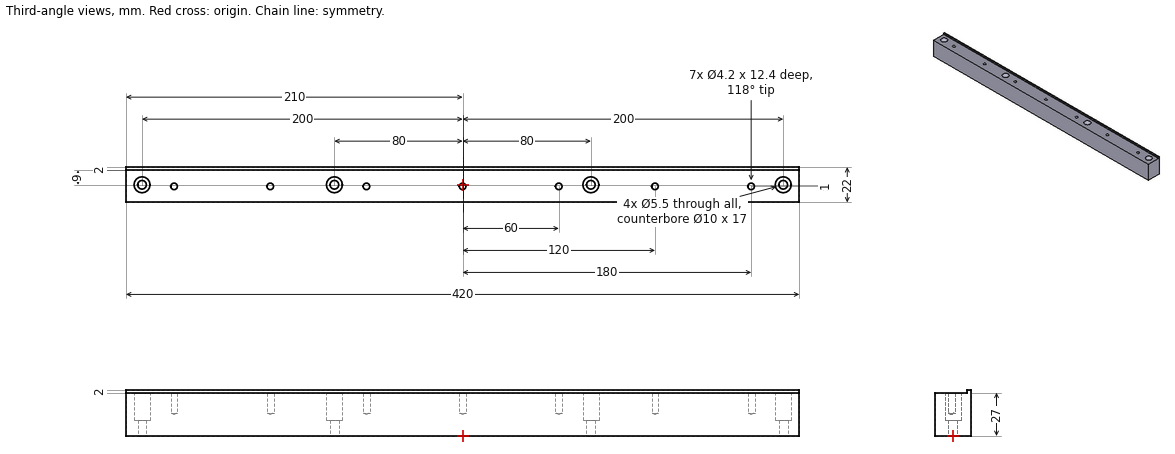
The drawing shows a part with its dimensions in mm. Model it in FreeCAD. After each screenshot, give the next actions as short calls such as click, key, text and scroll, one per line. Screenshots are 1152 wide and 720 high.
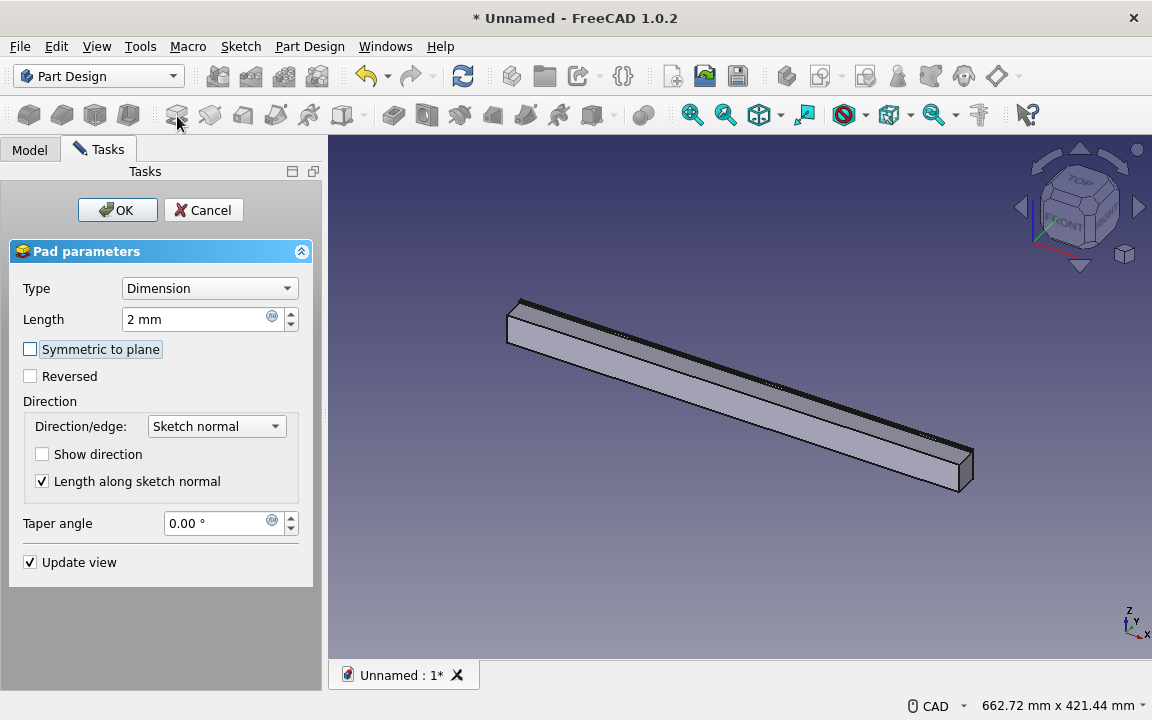
click(118, 210)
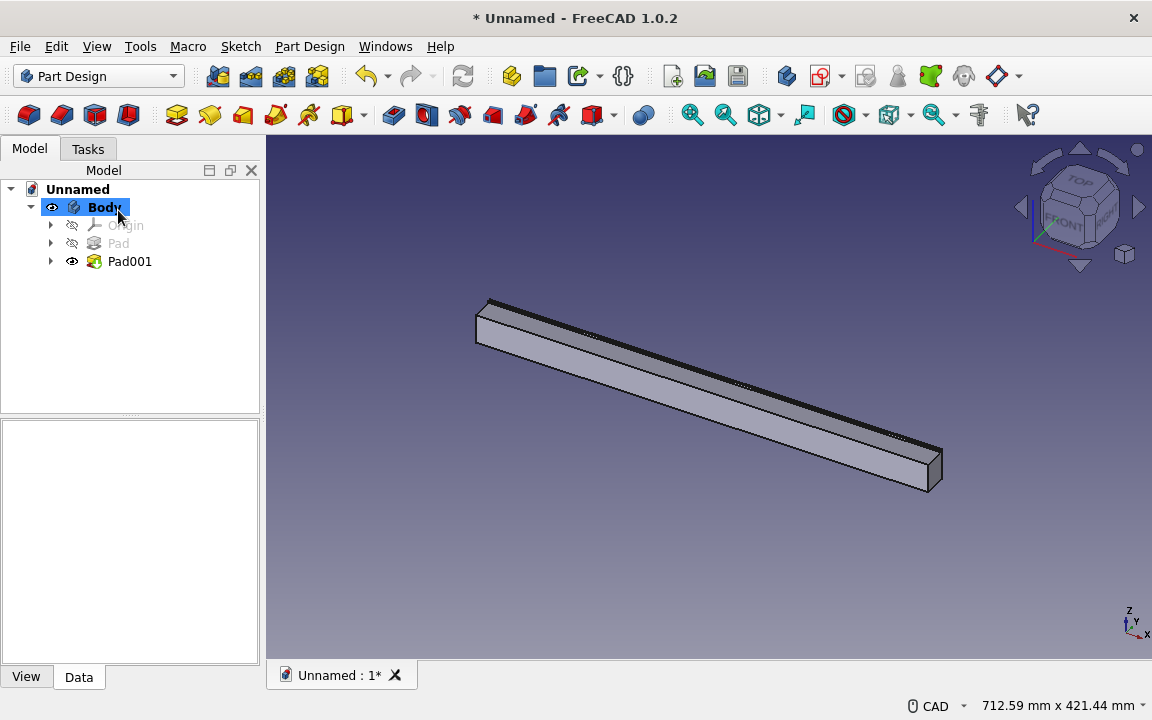
key(0)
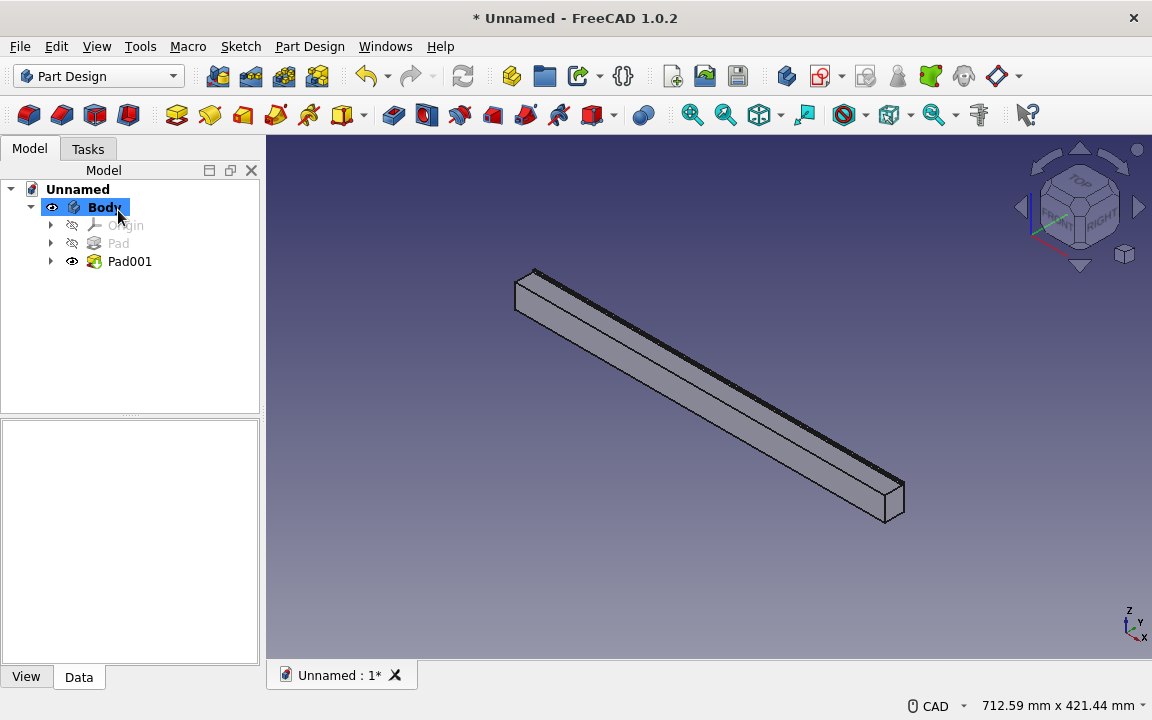
click(762, 413)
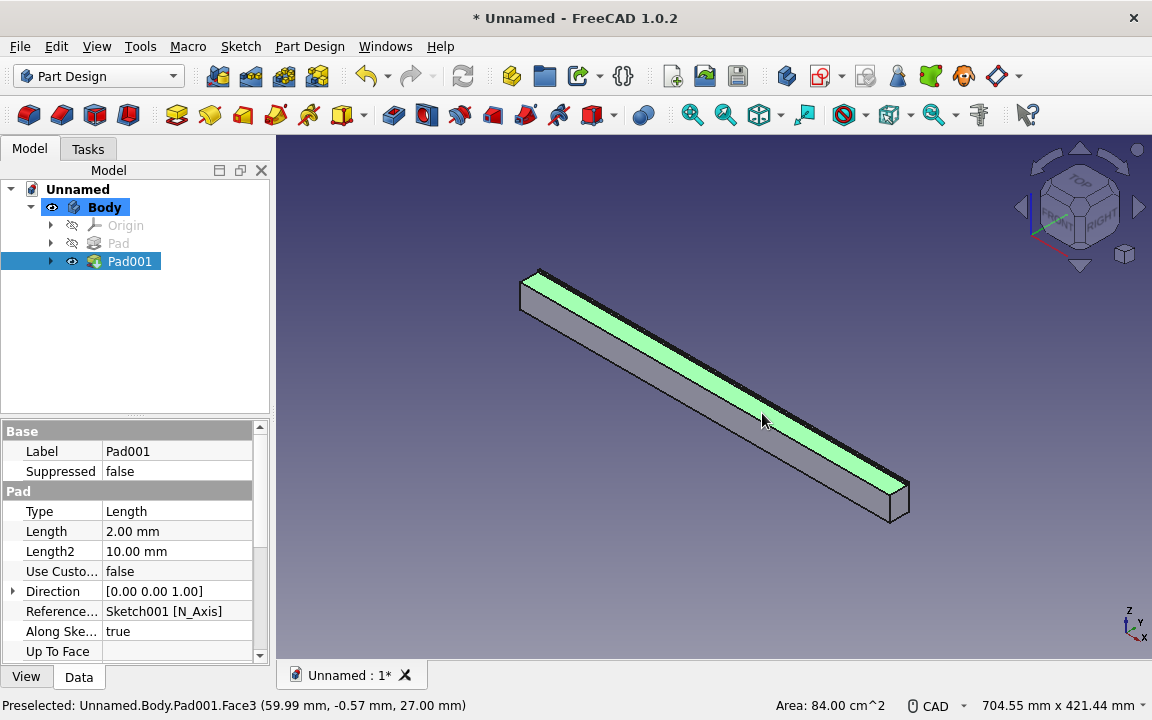
click(820, 76)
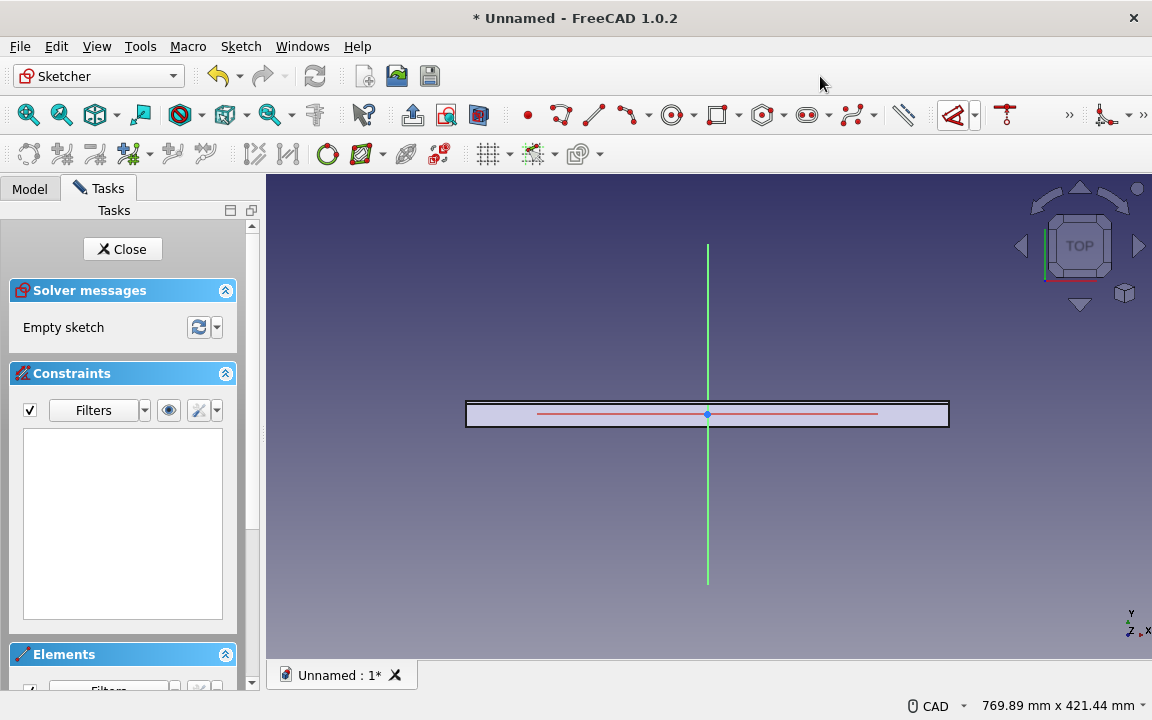
key(q)
key(s)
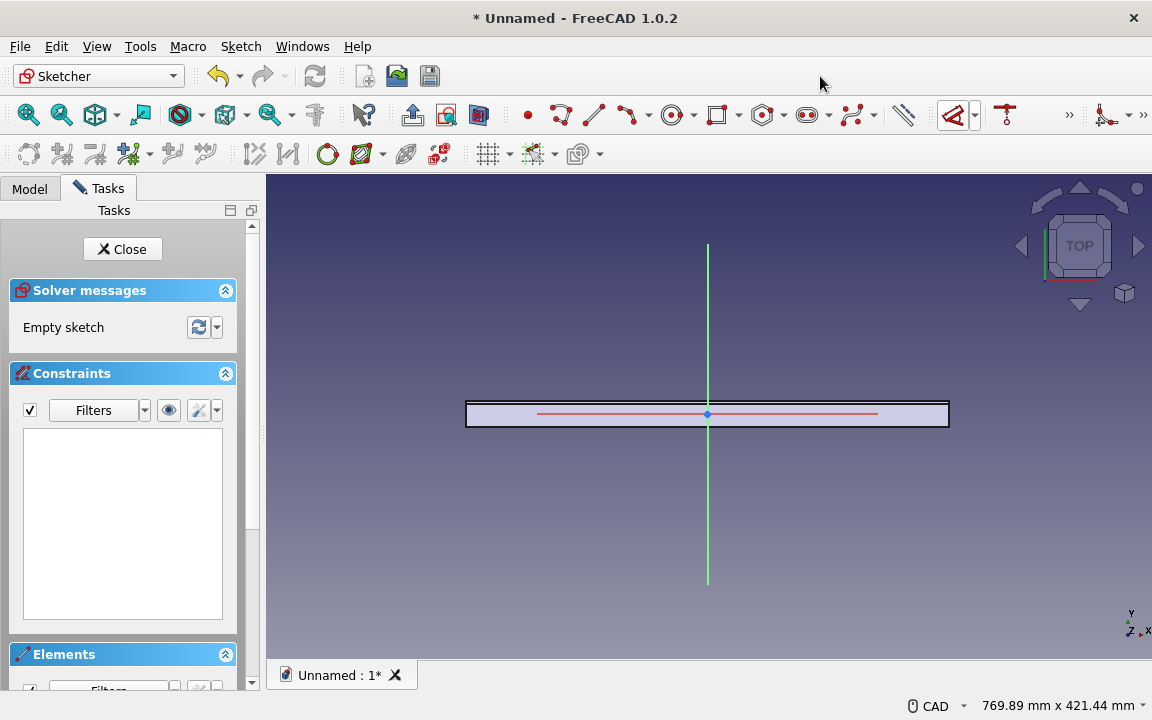
click(672, 116)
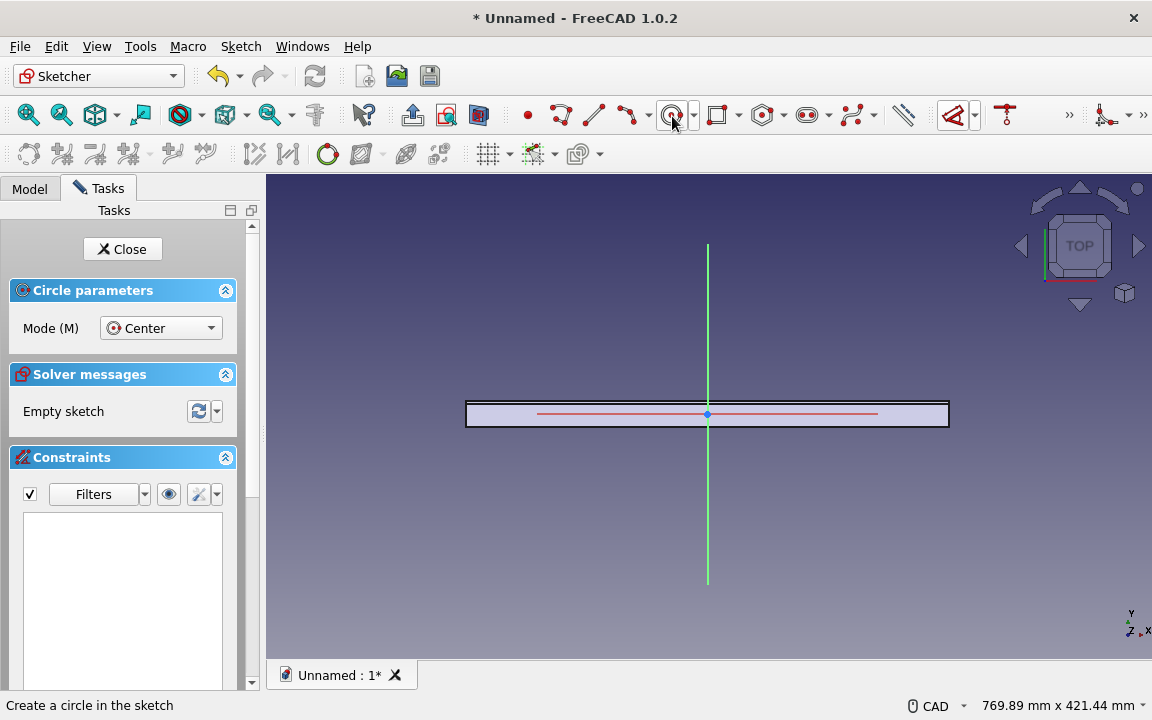
scroll(915, 415, up, 14)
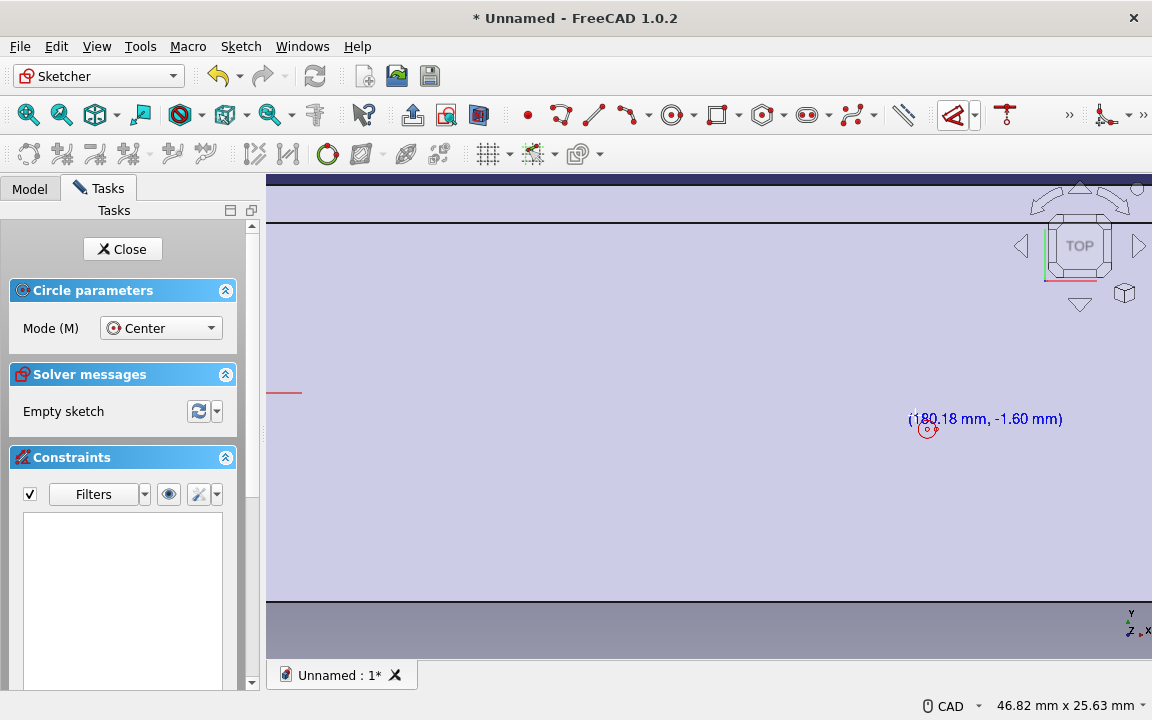
click(900, 412)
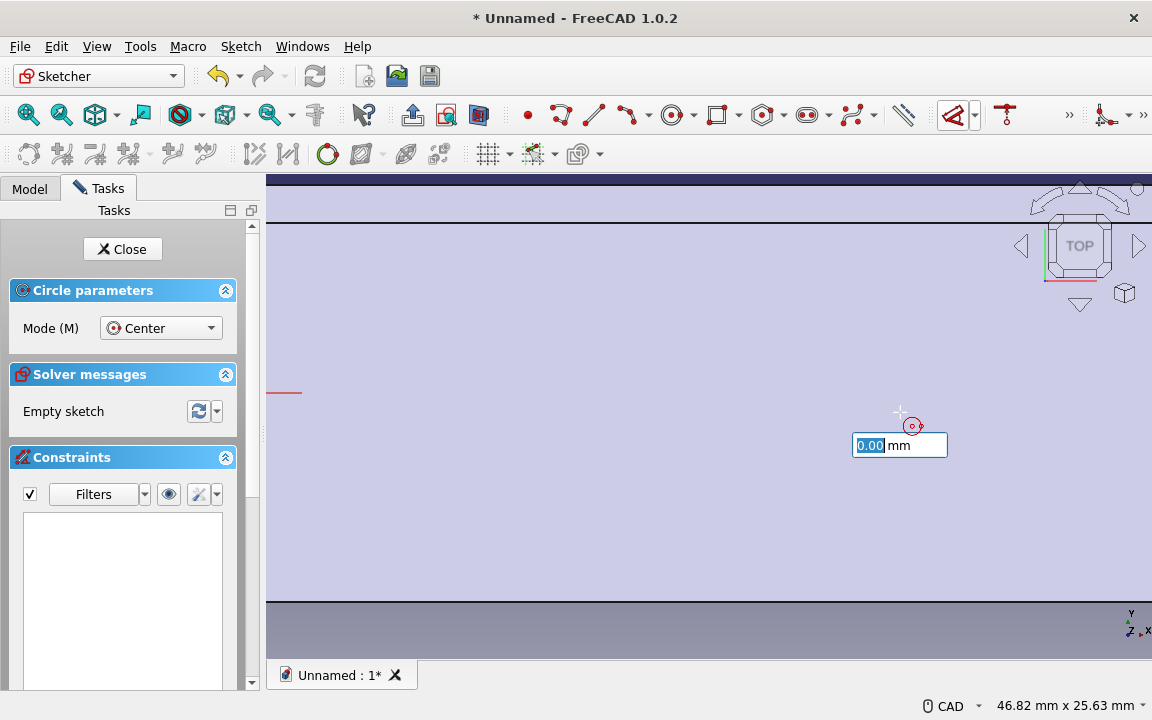
scroll(893, 417, down, 13)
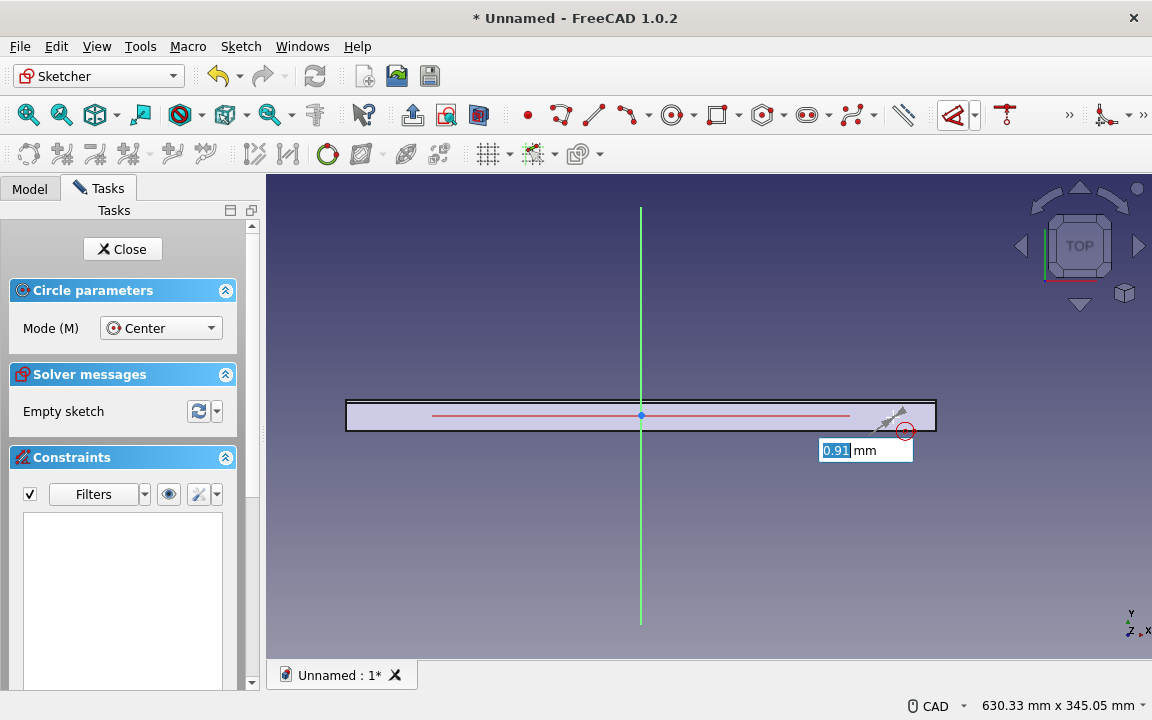
scroll(896, 419, up, 8)
move(895, 418)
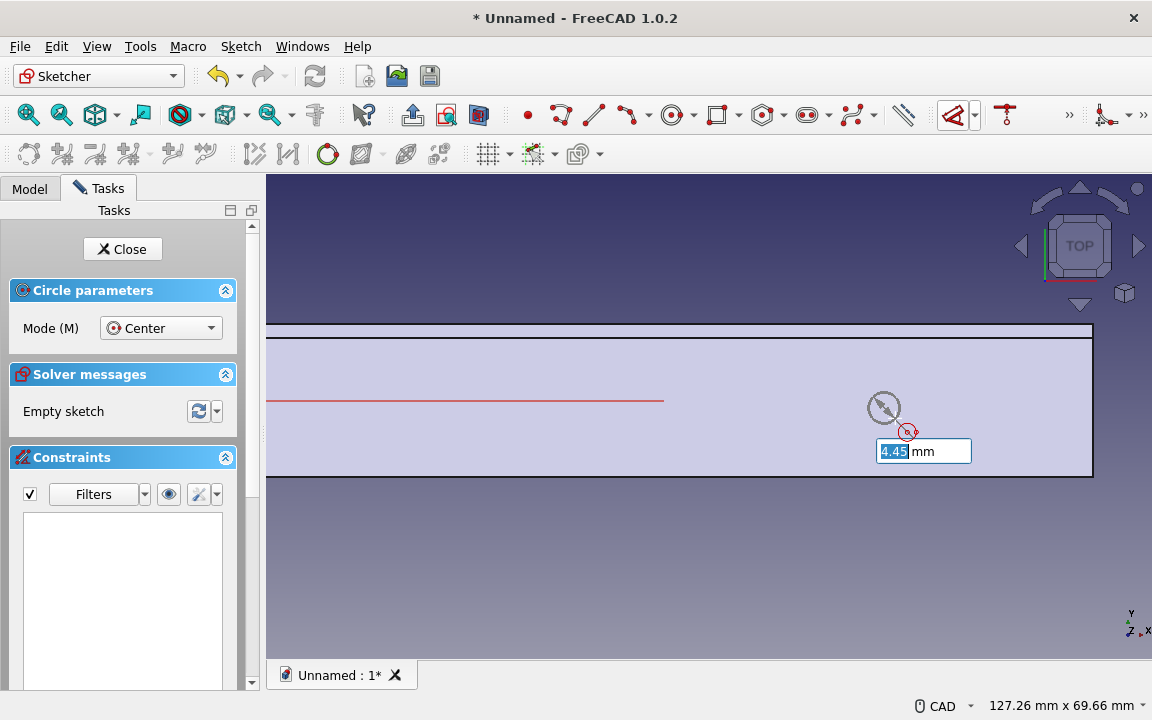
text(4.2)
key(Return)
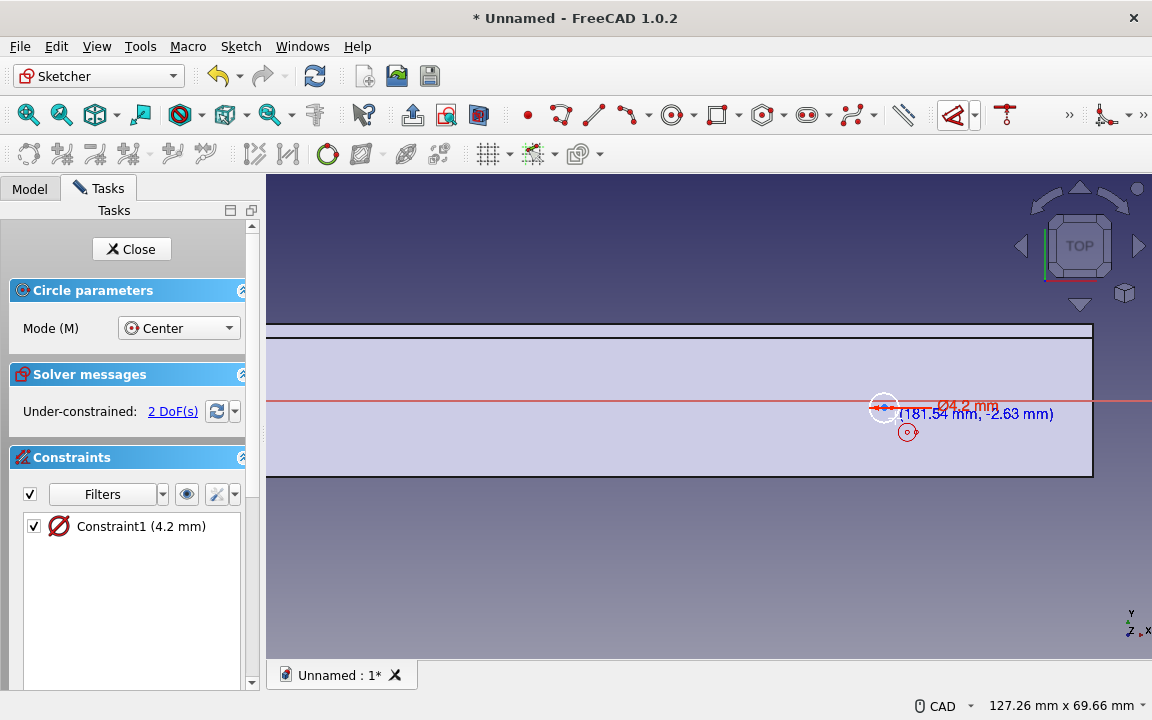
scroll(467, 408, up, 5)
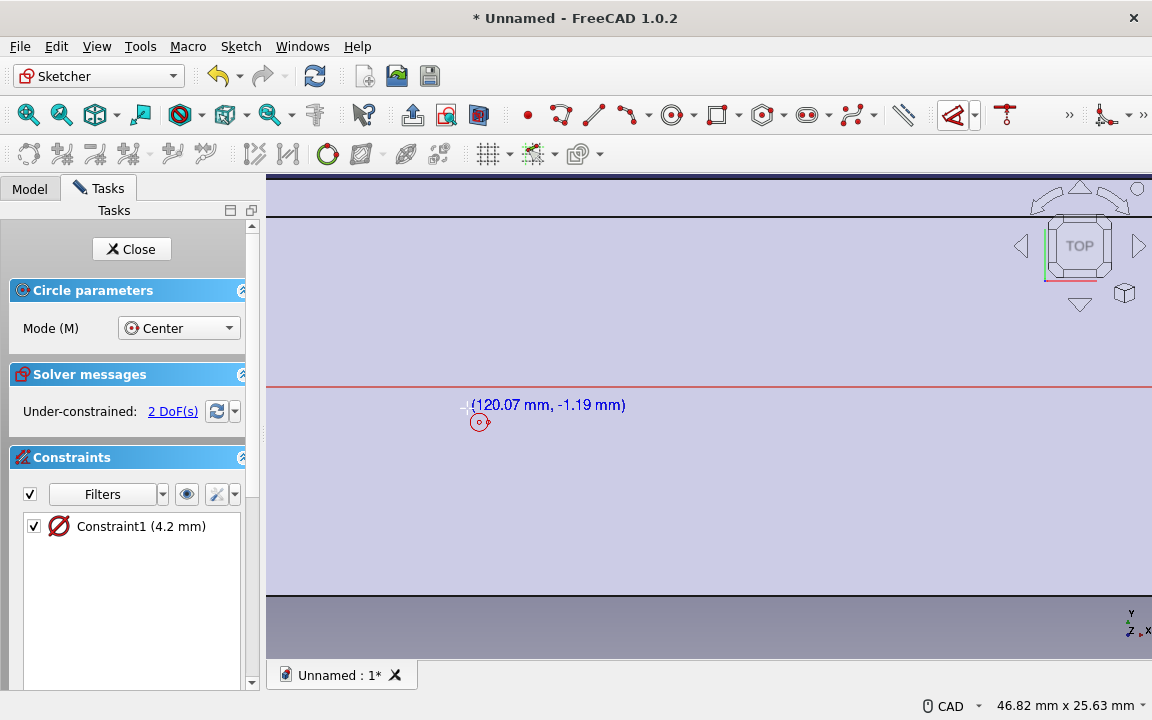
click(465, 406)